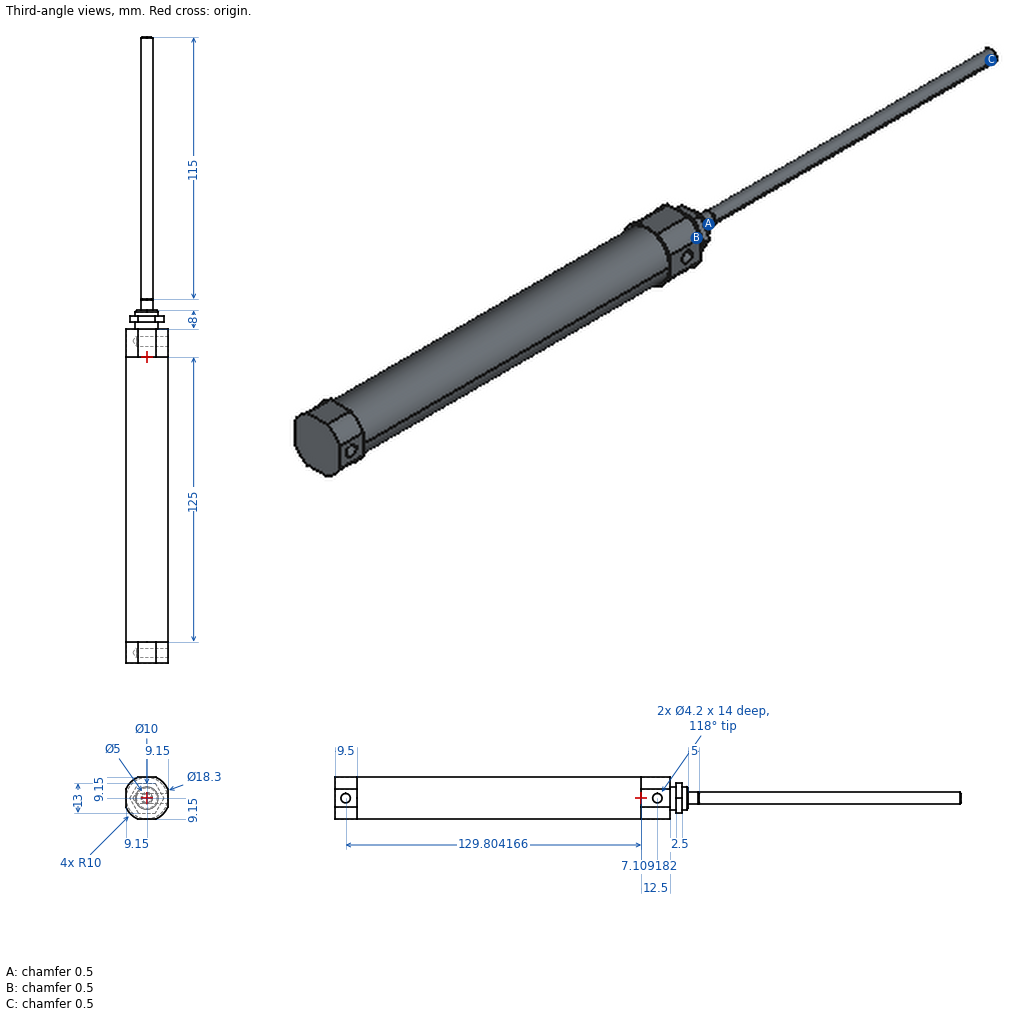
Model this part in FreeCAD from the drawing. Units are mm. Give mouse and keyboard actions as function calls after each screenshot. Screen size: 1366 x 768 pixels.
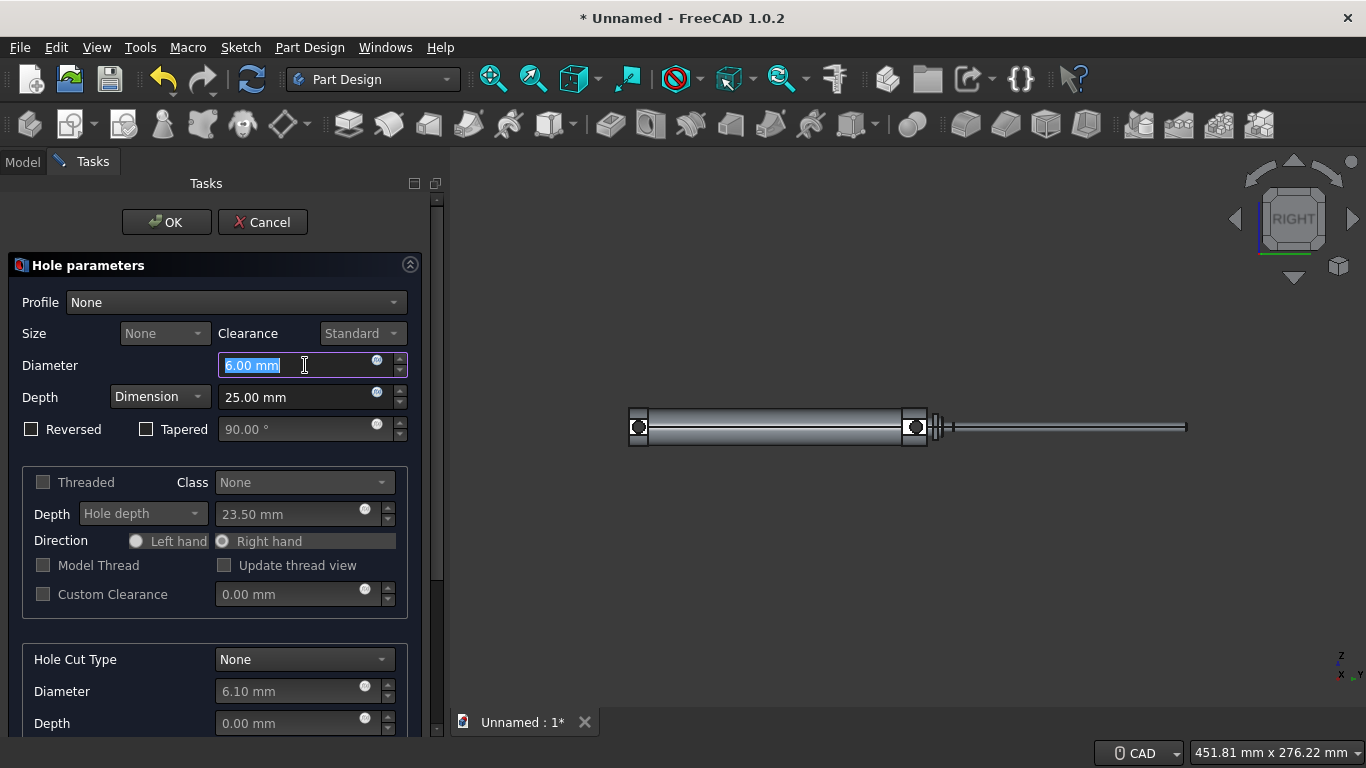
text(4.2)
key(Tab)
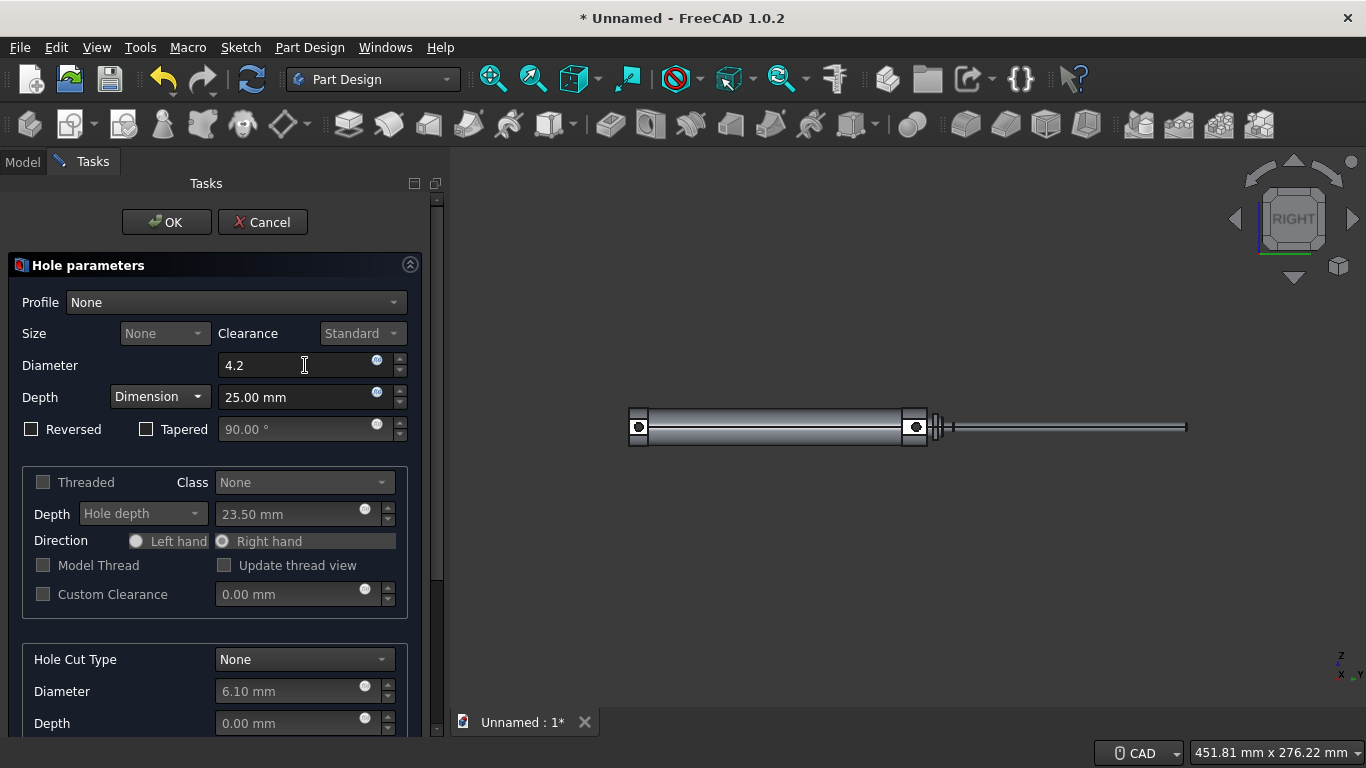
triple_click(305, 397)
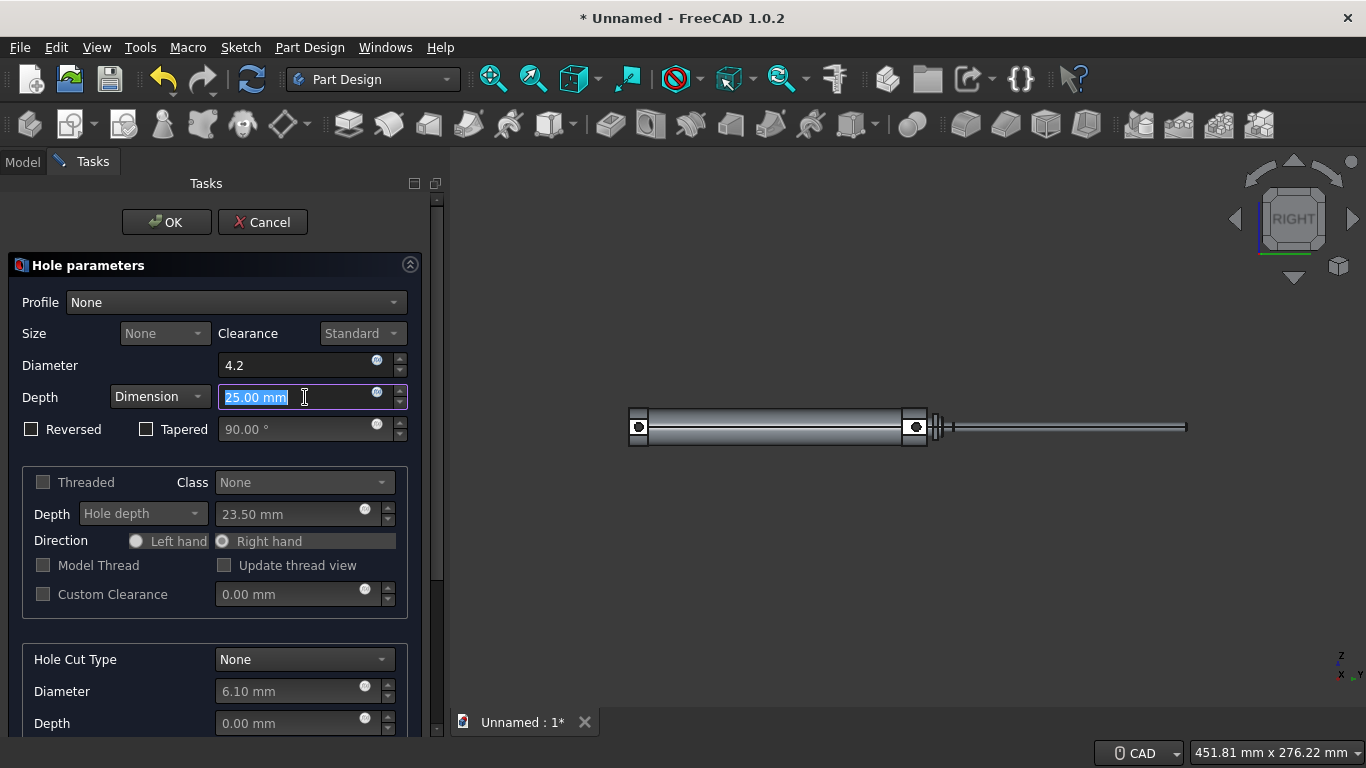
text(14)
key(Tab)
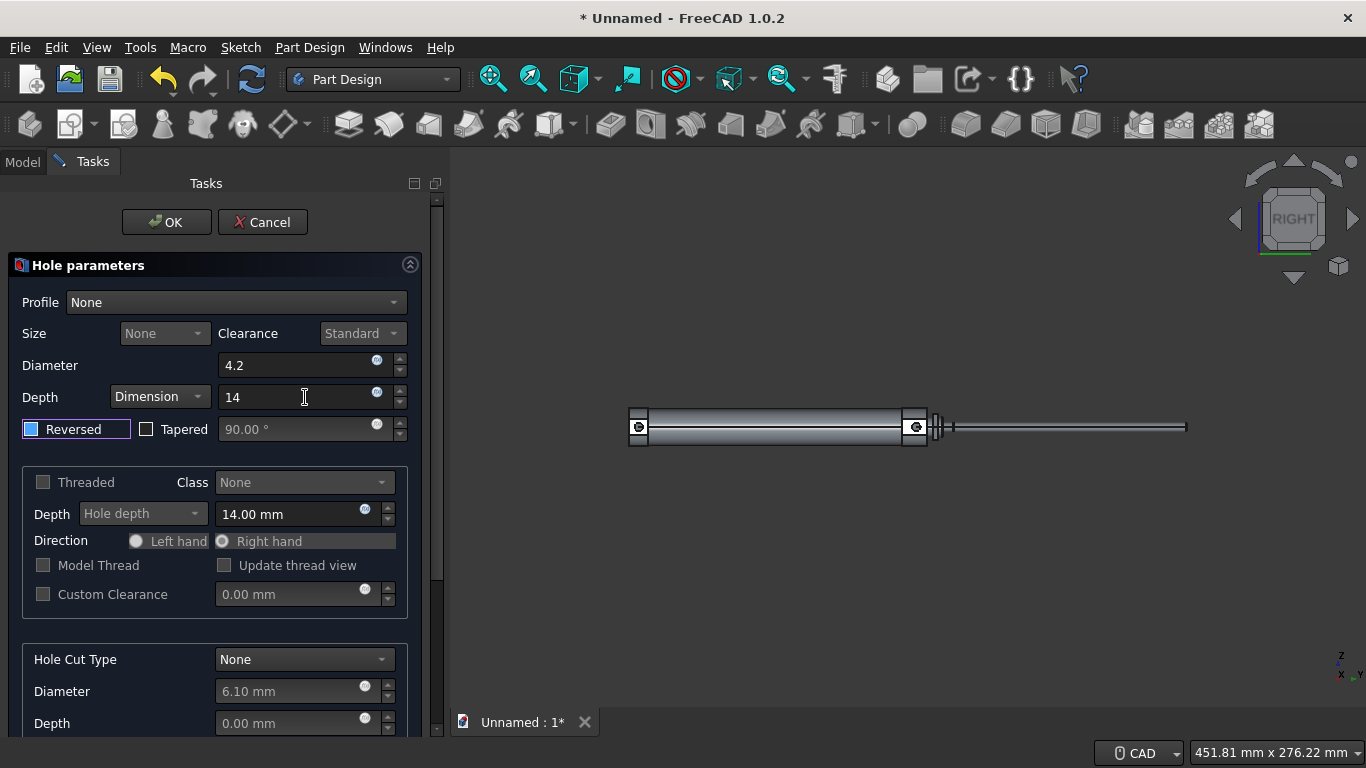
click(167, 222)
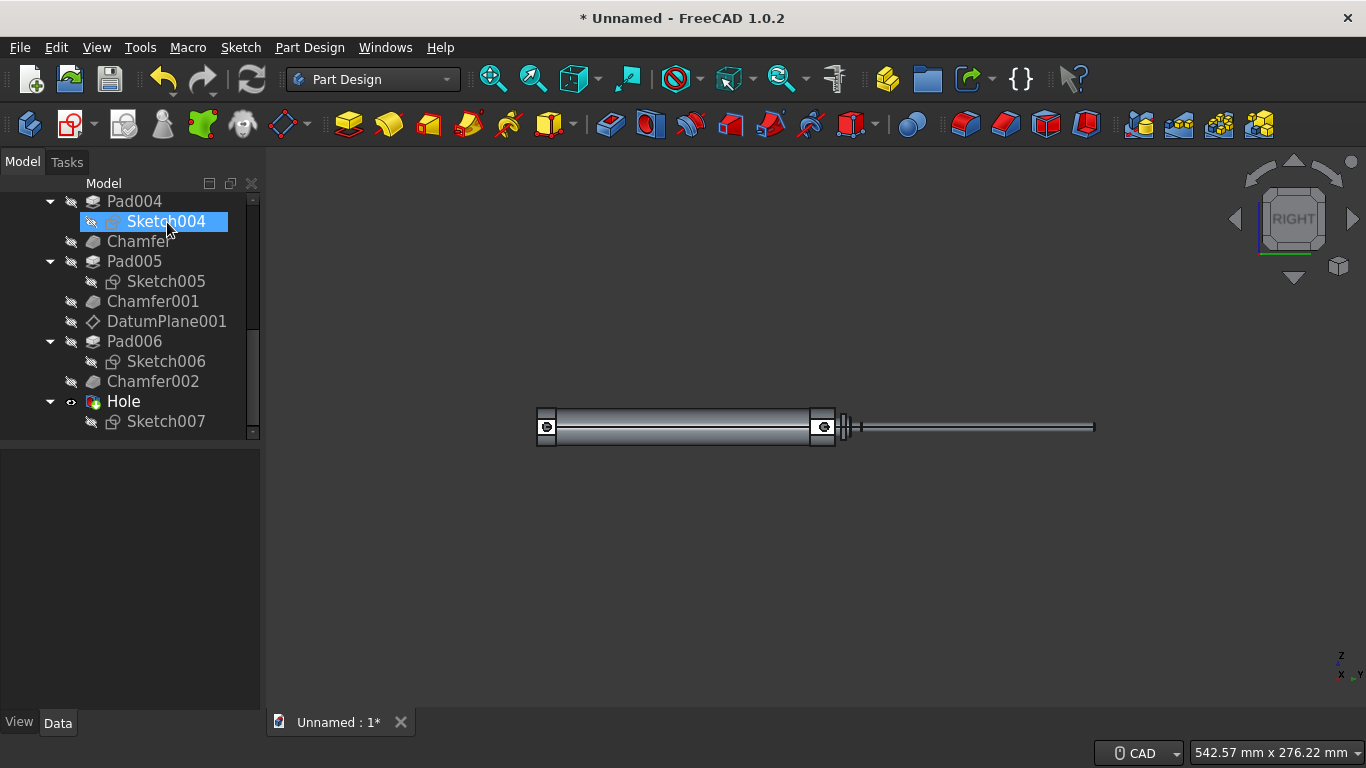
key(0)